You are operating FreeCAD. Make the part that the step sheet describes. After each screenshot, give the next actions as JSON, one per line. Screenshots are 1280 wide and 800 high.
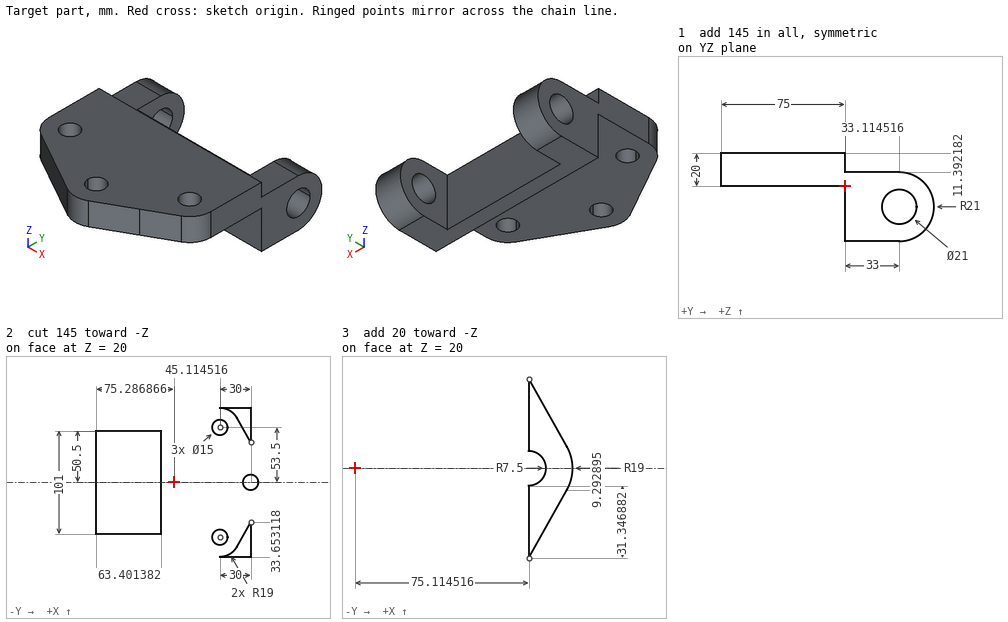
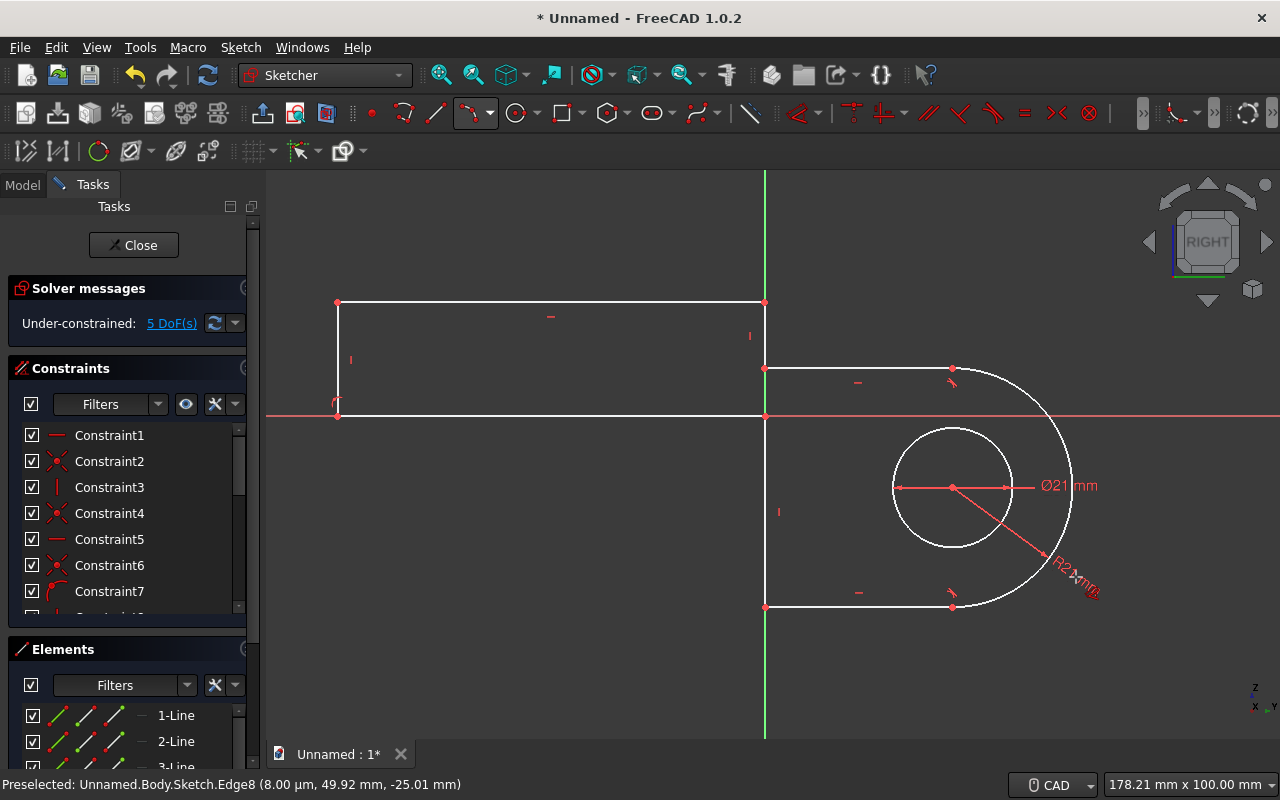
{"action": "left_click", "coordinate": [637, 302]}
{"action": "left_click", "coordinate": [551, 268]}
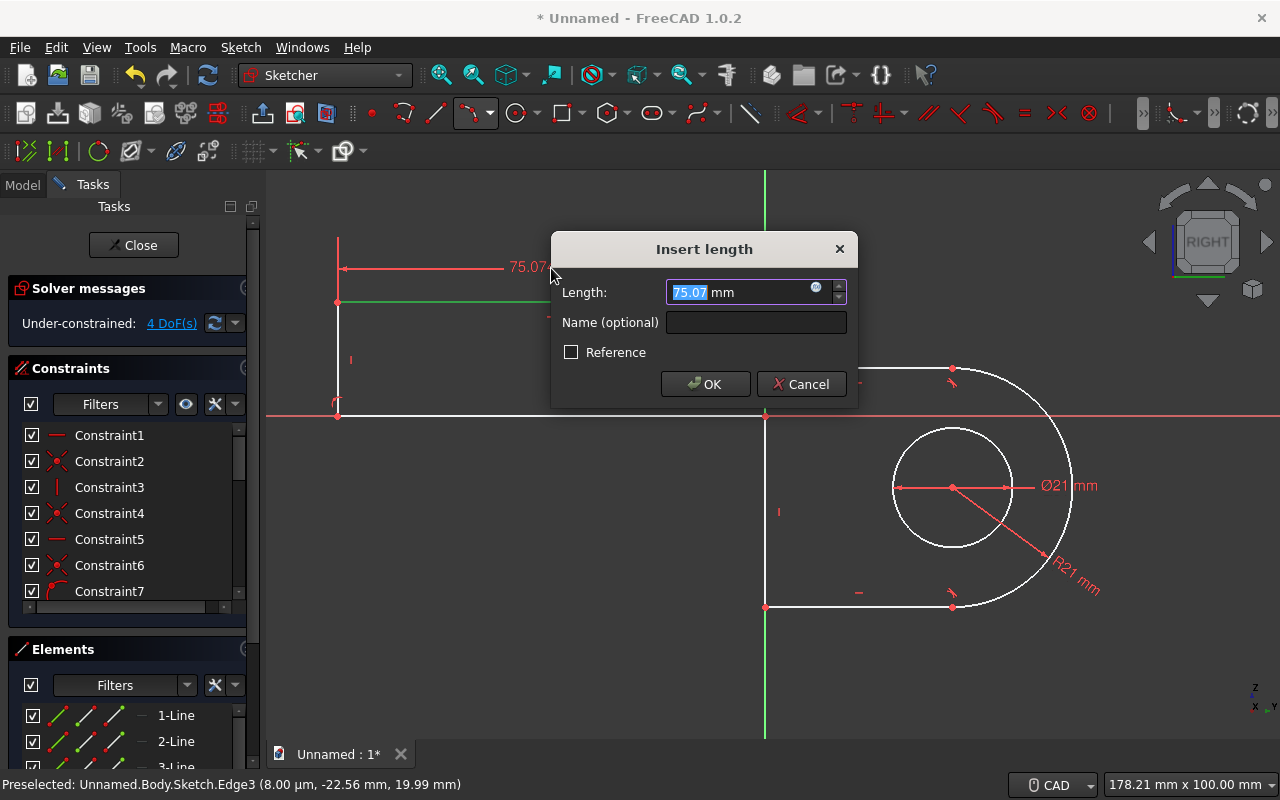
{"action": "type", "text": "75"}
{"action": "key", "text": "Return"}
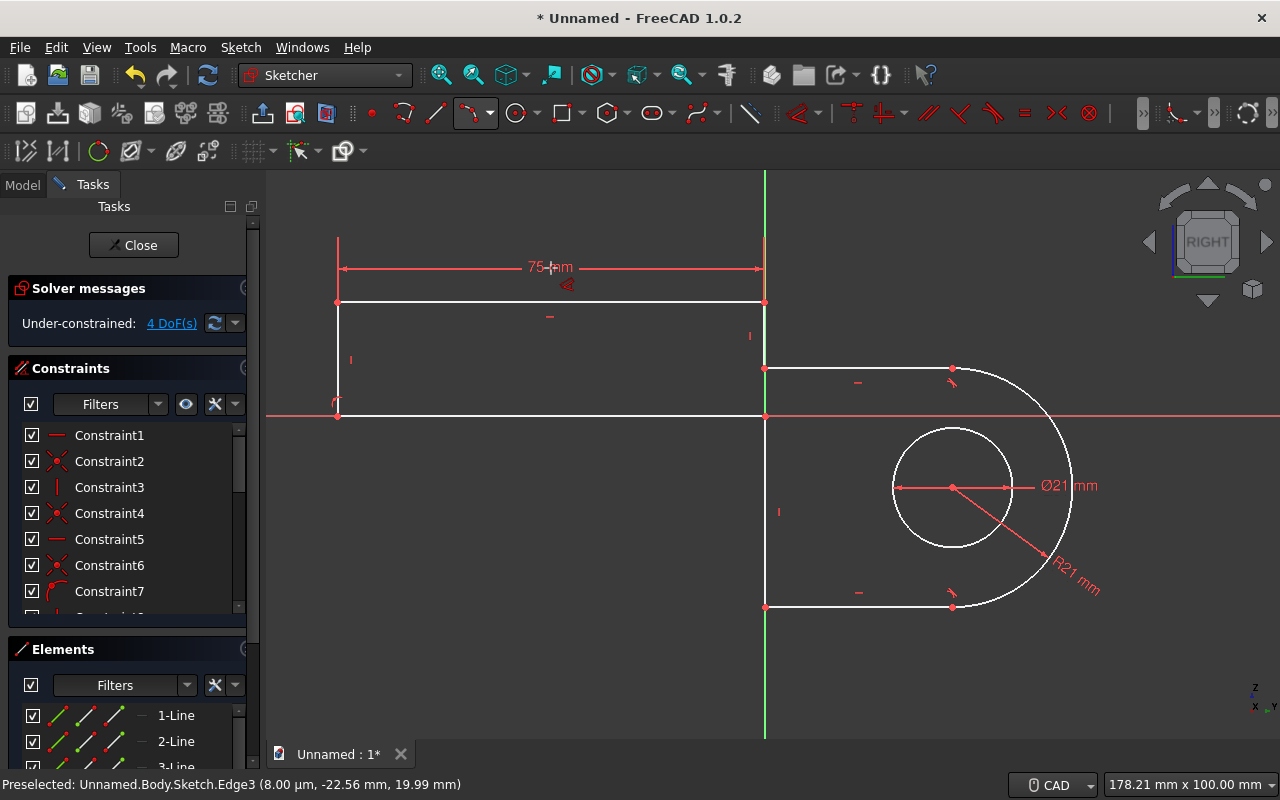
{"action": "left_click", "coordinate": [338, 337]}
{"action": "left_click", "coordinate": [304, 359]}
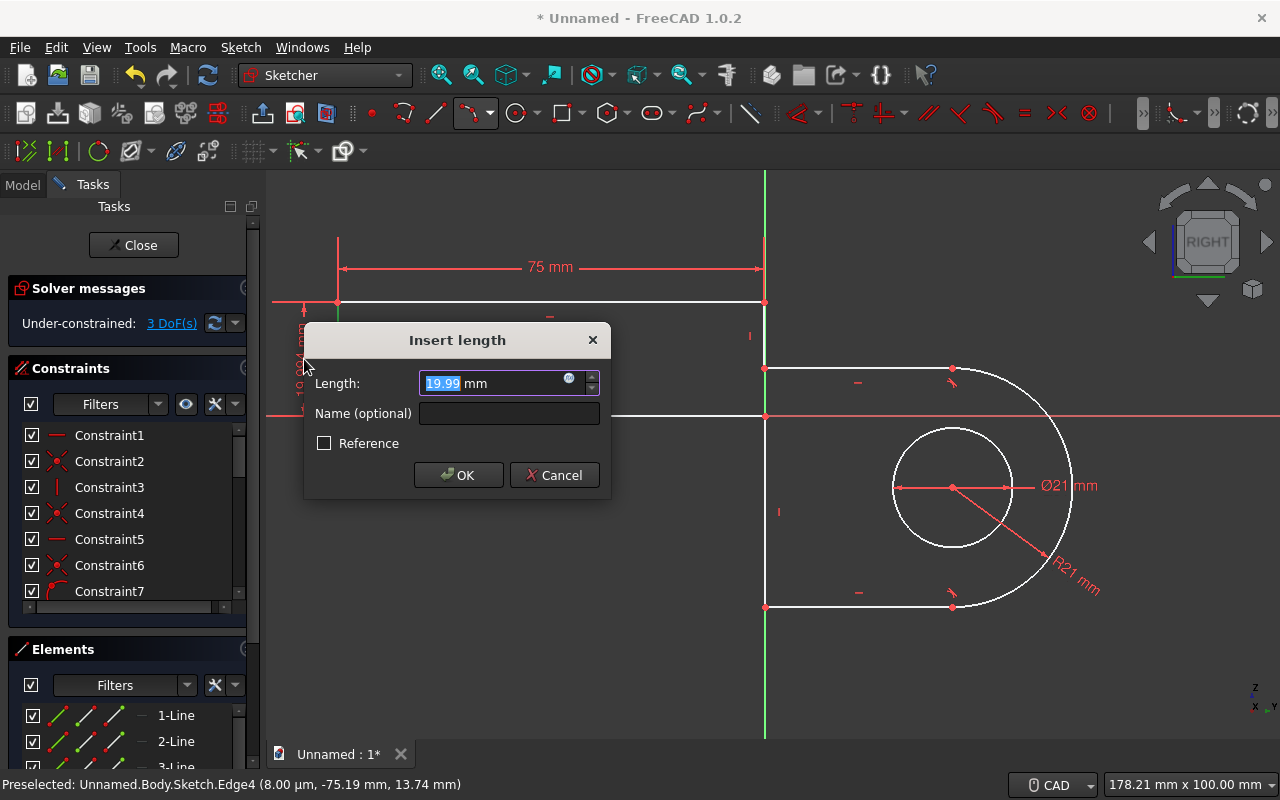
{"action": "type", "text": "20"}
{"action": "key", "text": "Return"}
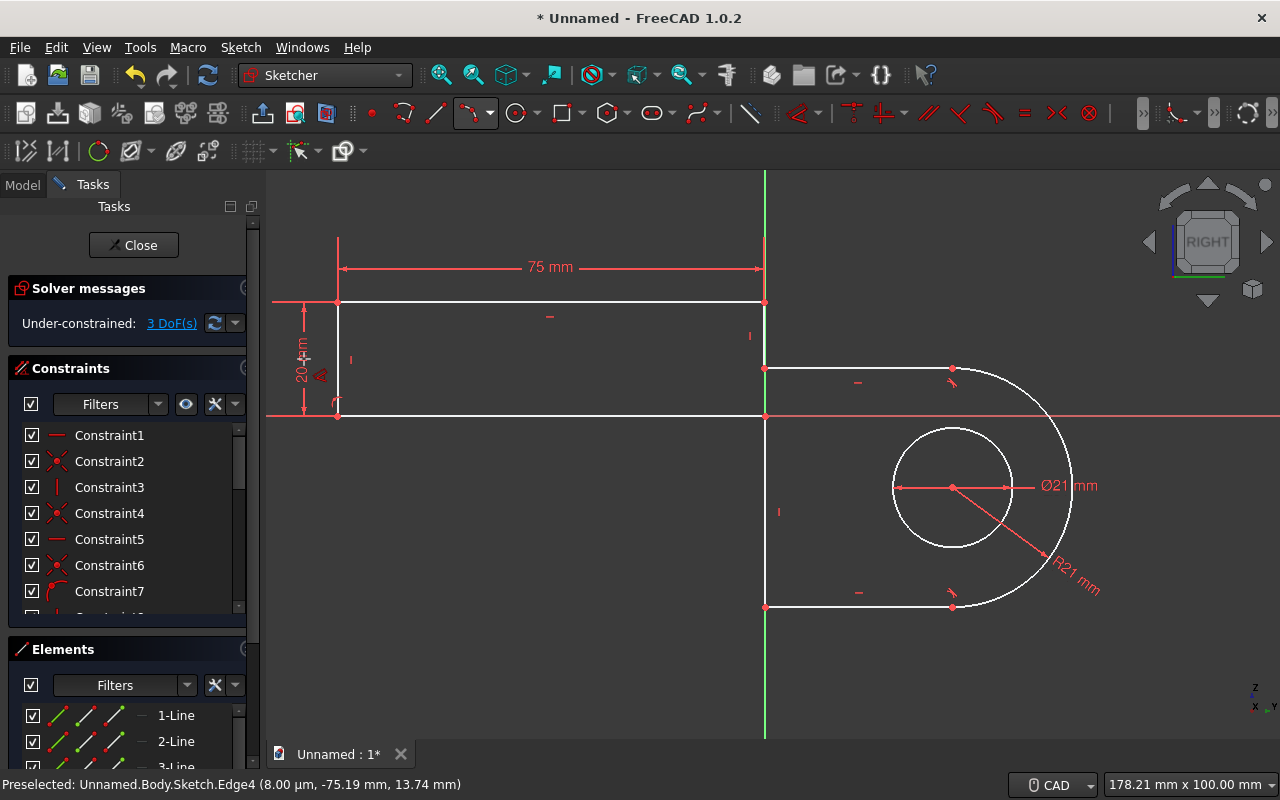
{"action": "left_click", "coordinate": [822, 607]}
{"action": "left_click", "coordinate": [859, 641]}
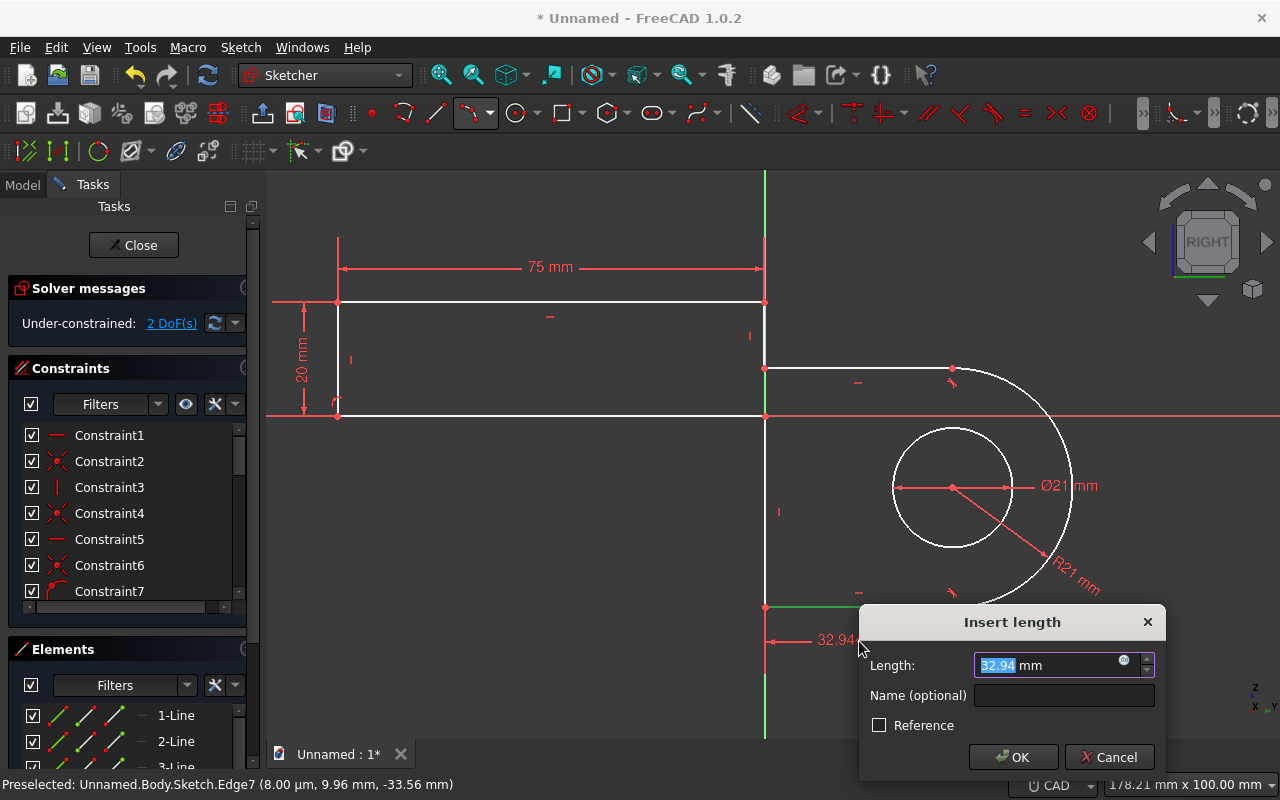
{"action": "type", "text": "33"}
{"action": "key", "text": "Return"}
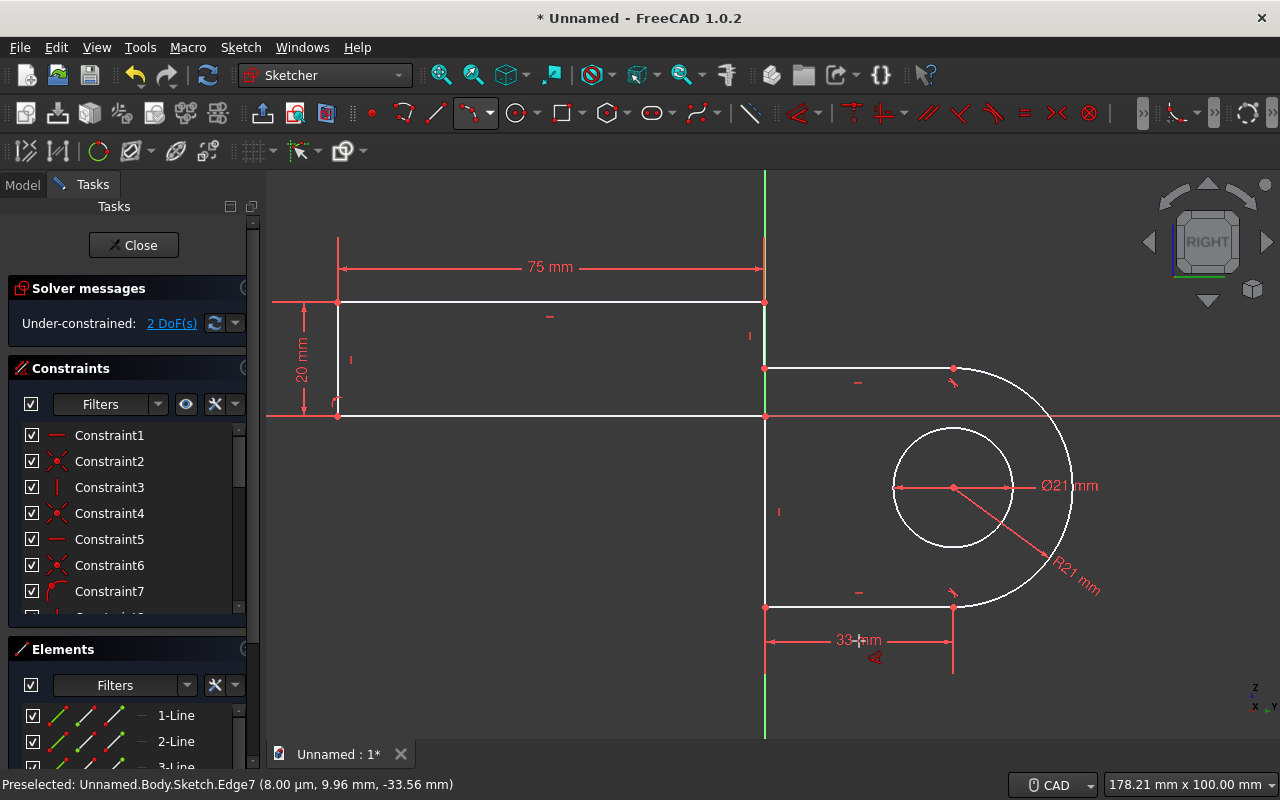
{"action": "left_click", "coordinate": [896, 368]}
{"action": "left_click", "coordinate": [859, 334]}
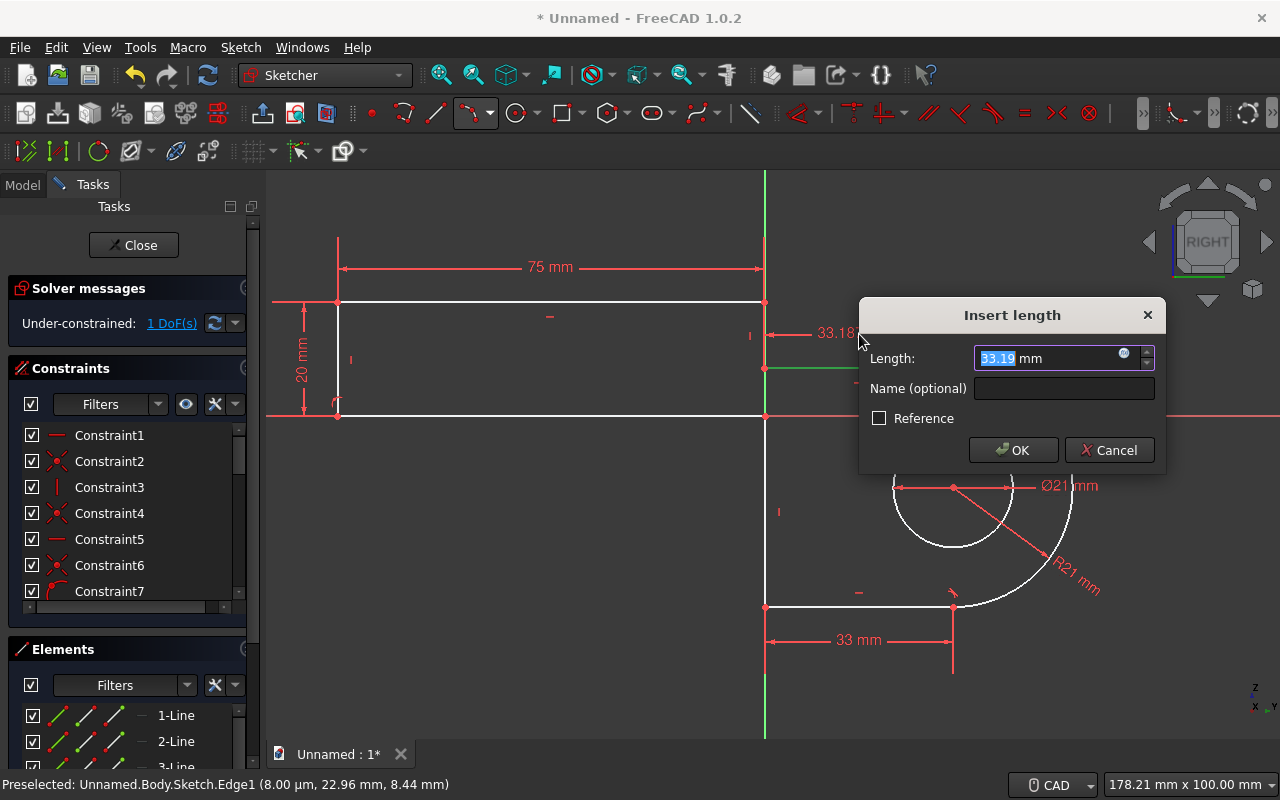
{"action": "type", "text": "33.114516"}
{"action": "key", "text": "Return"}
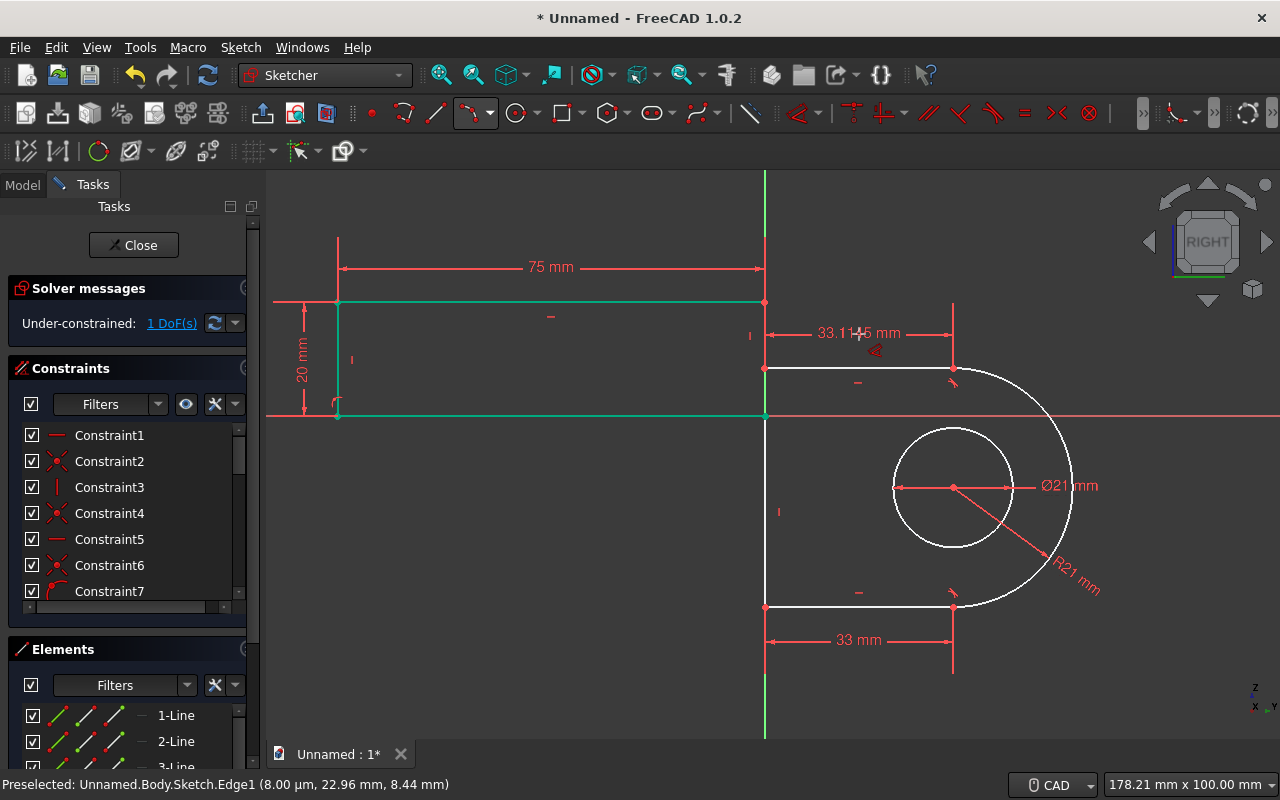
{"action": "left_click", "coordinate": [765, 348]}
{"action": "left_click", "coordinate": [799, 312]}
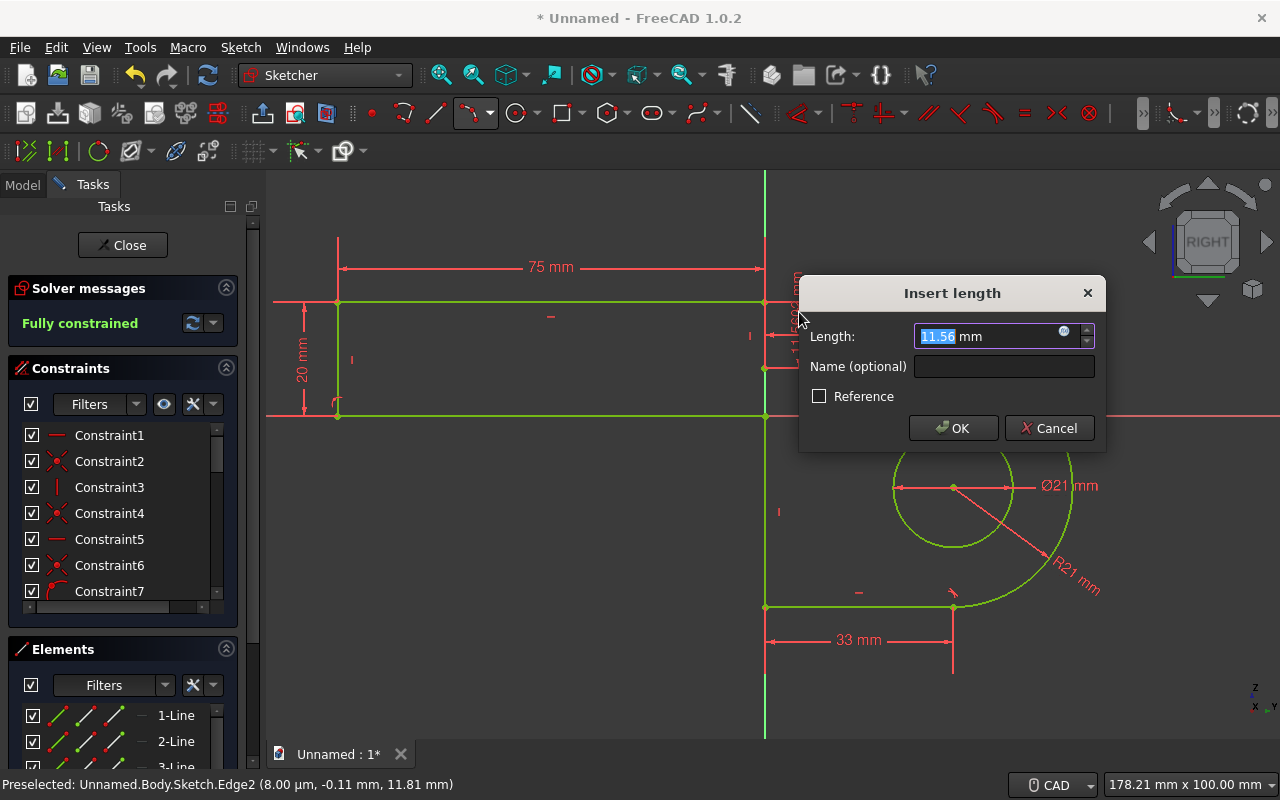
{"action": "type", "text": "11.392182"}
{"action": "key", "text": "Return"}
{"action": "key", "text": "Escape"}